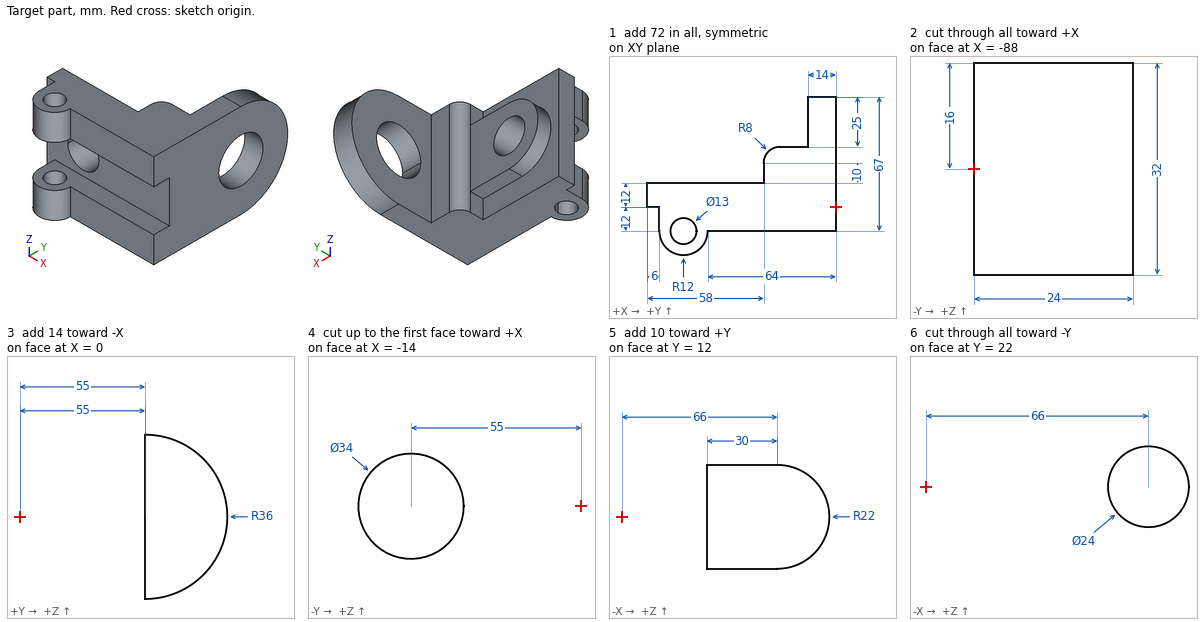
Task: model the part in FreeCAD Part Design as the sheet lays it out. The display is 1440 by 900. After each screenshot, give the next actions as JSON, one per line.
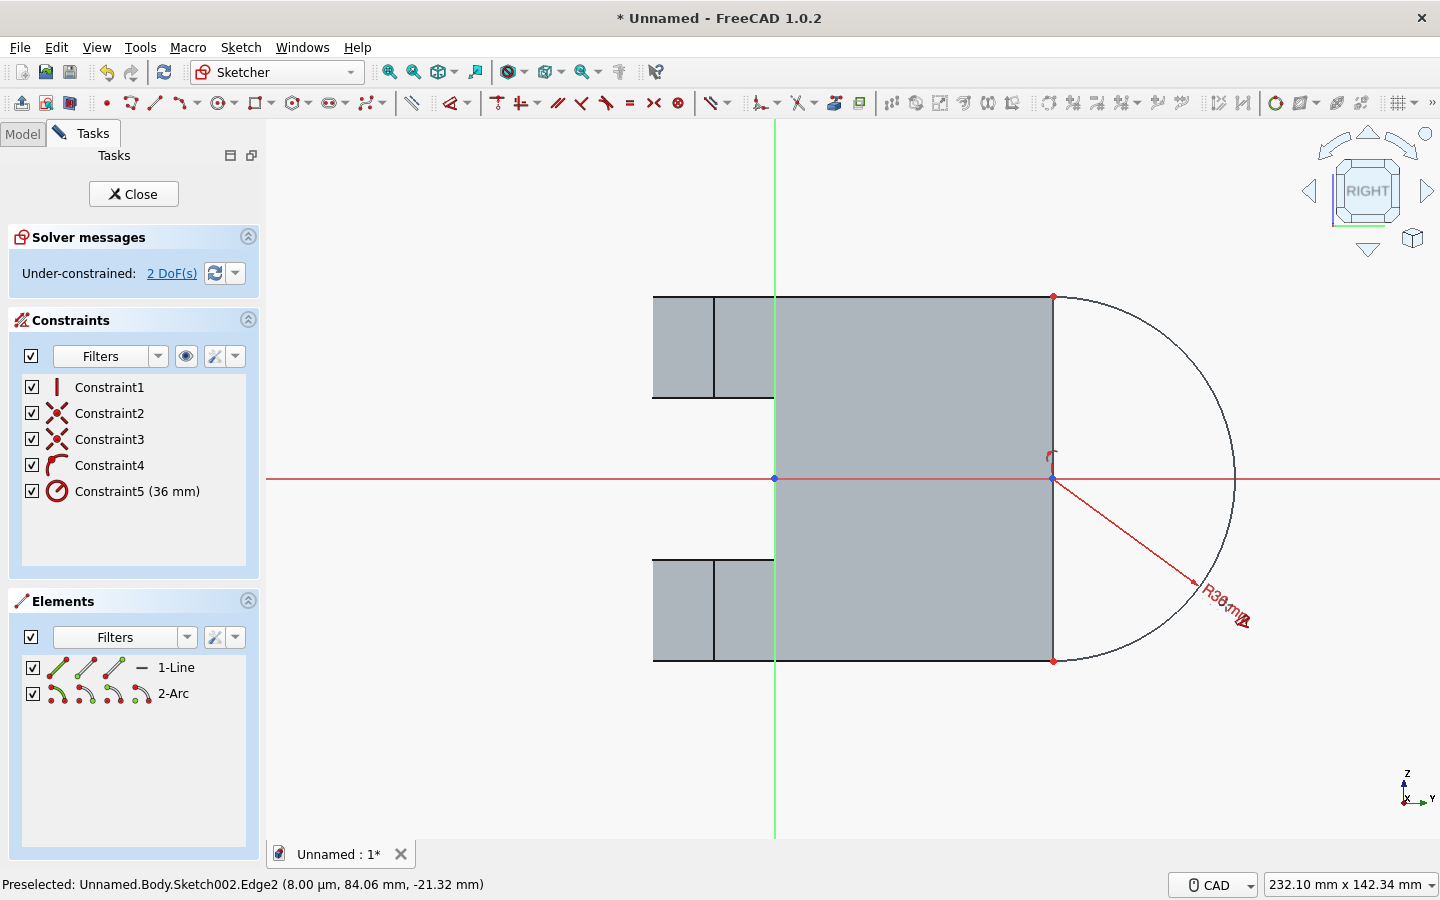
{"action": "left_click", "coordinate": [1053, 297]}
{"action": "left_click", "coordinate": [914, 263]}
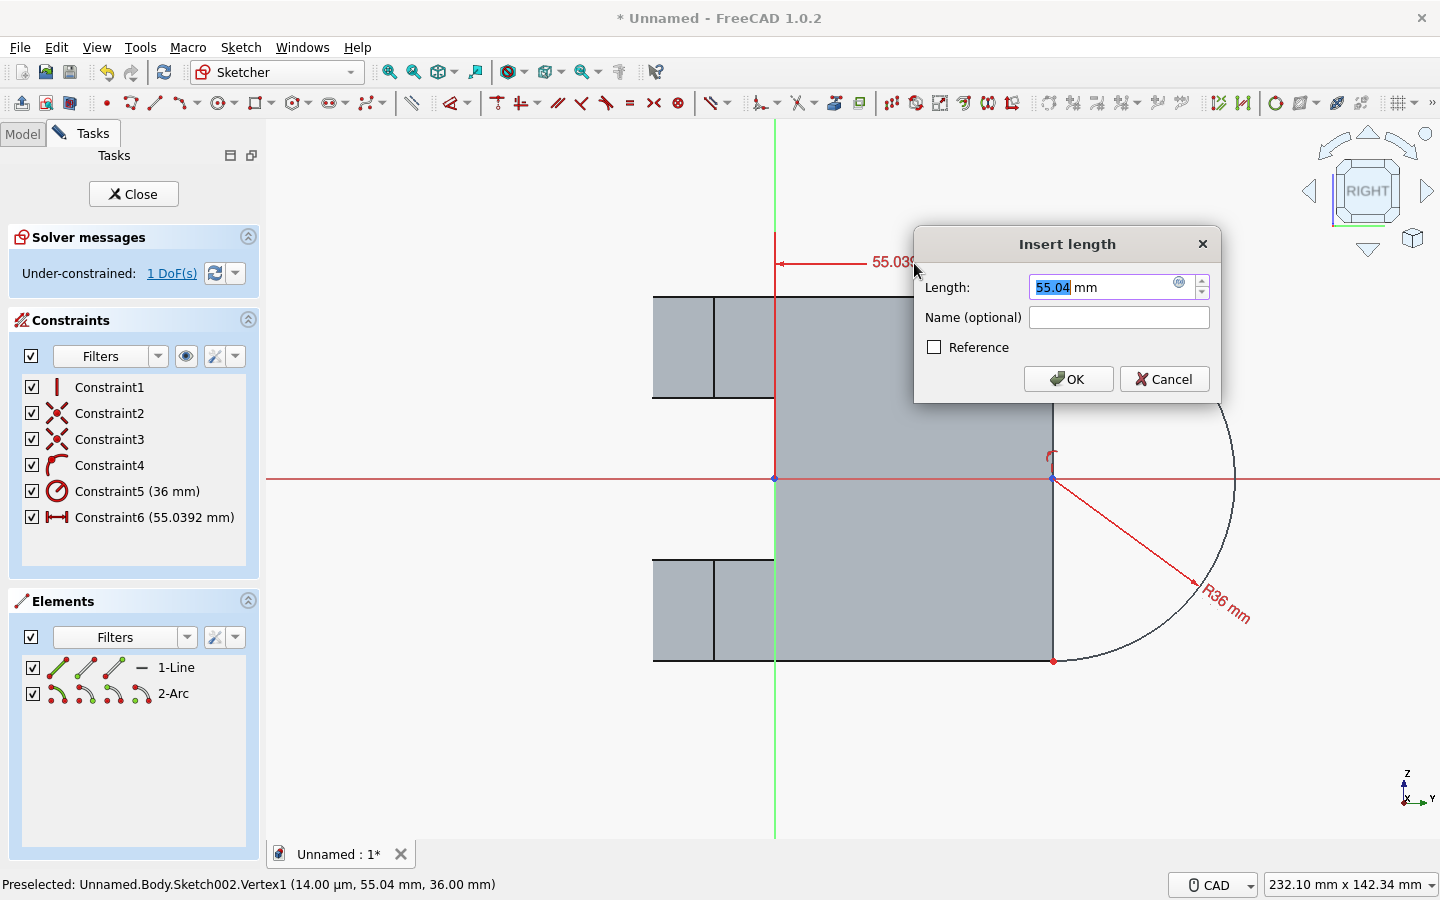
{"action": "type", "text": "55"}
{"action": "key", "text": "Return"}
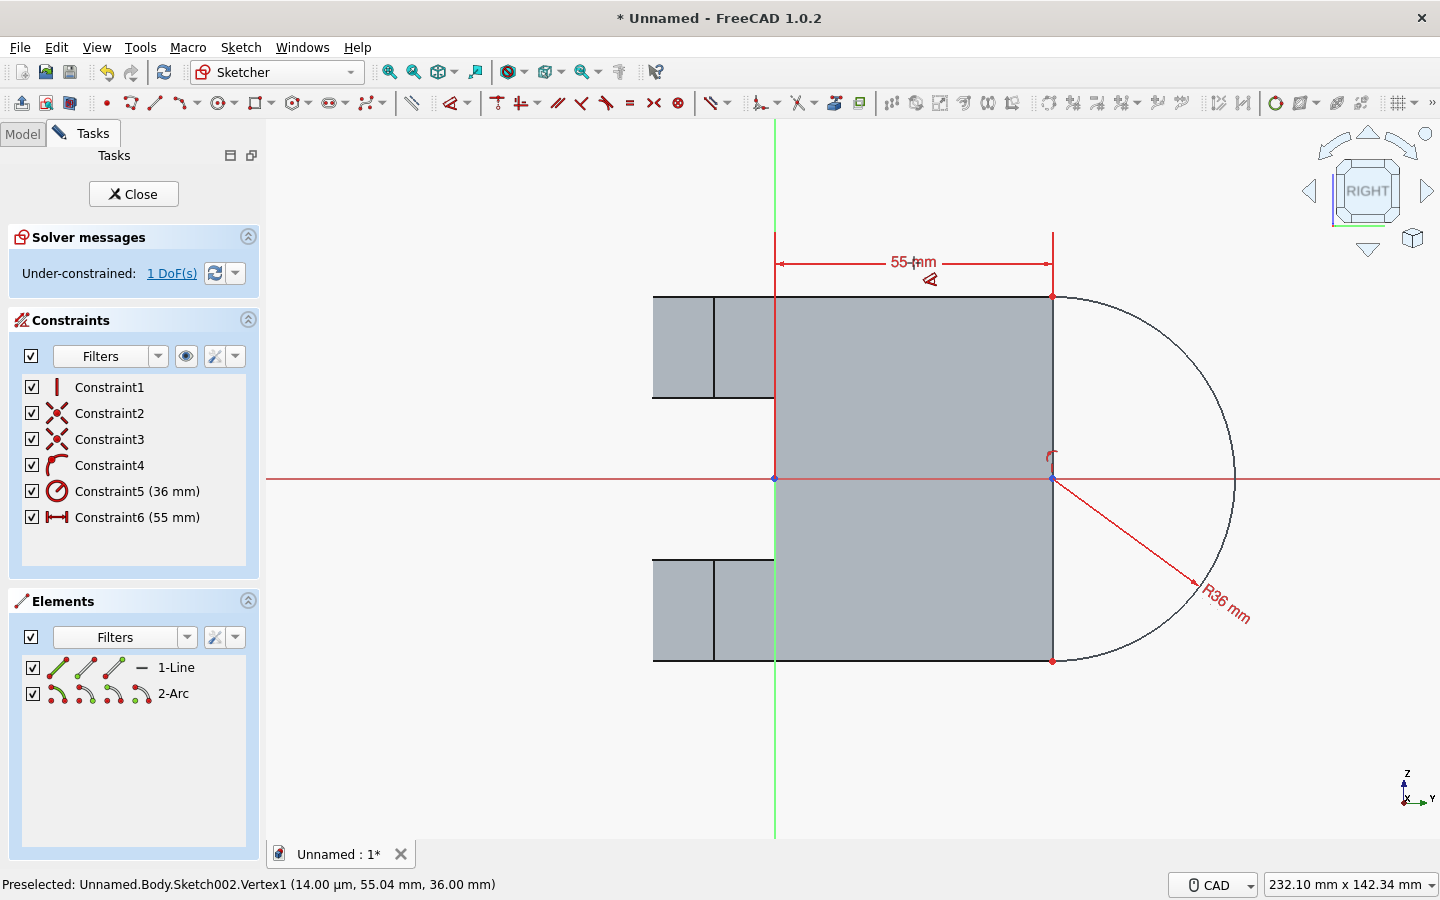
{"action": "left_click", "coordinate": [1053, 479]}
{"action": "left_click", "coordinate": [914, 513]}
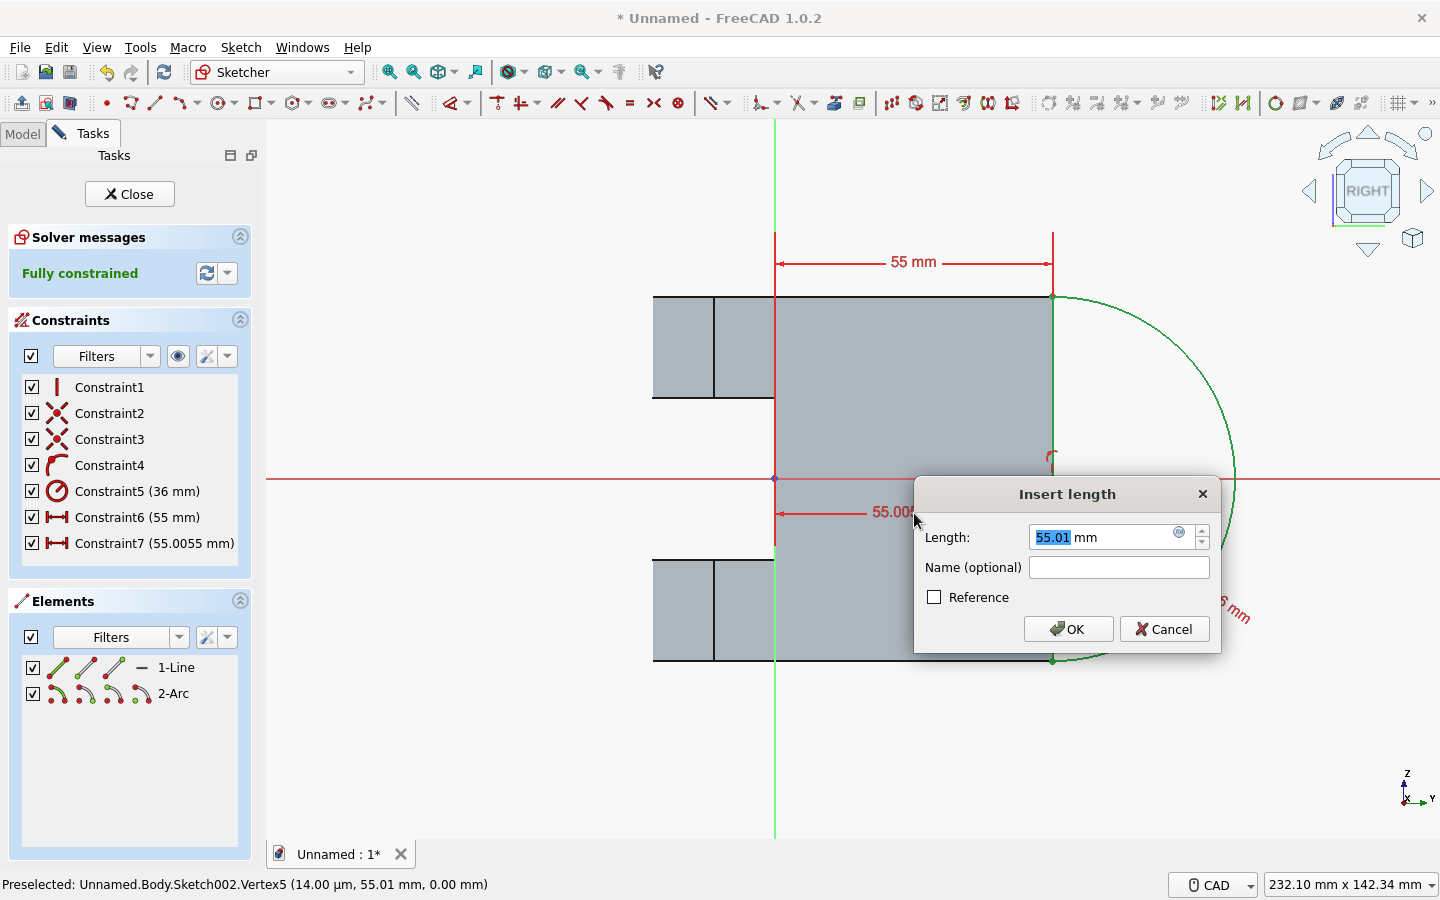
{"action": "type", "text": "55"}
{"action": "key", "text": "Return"}
{"action": "key", "text": "Escape"}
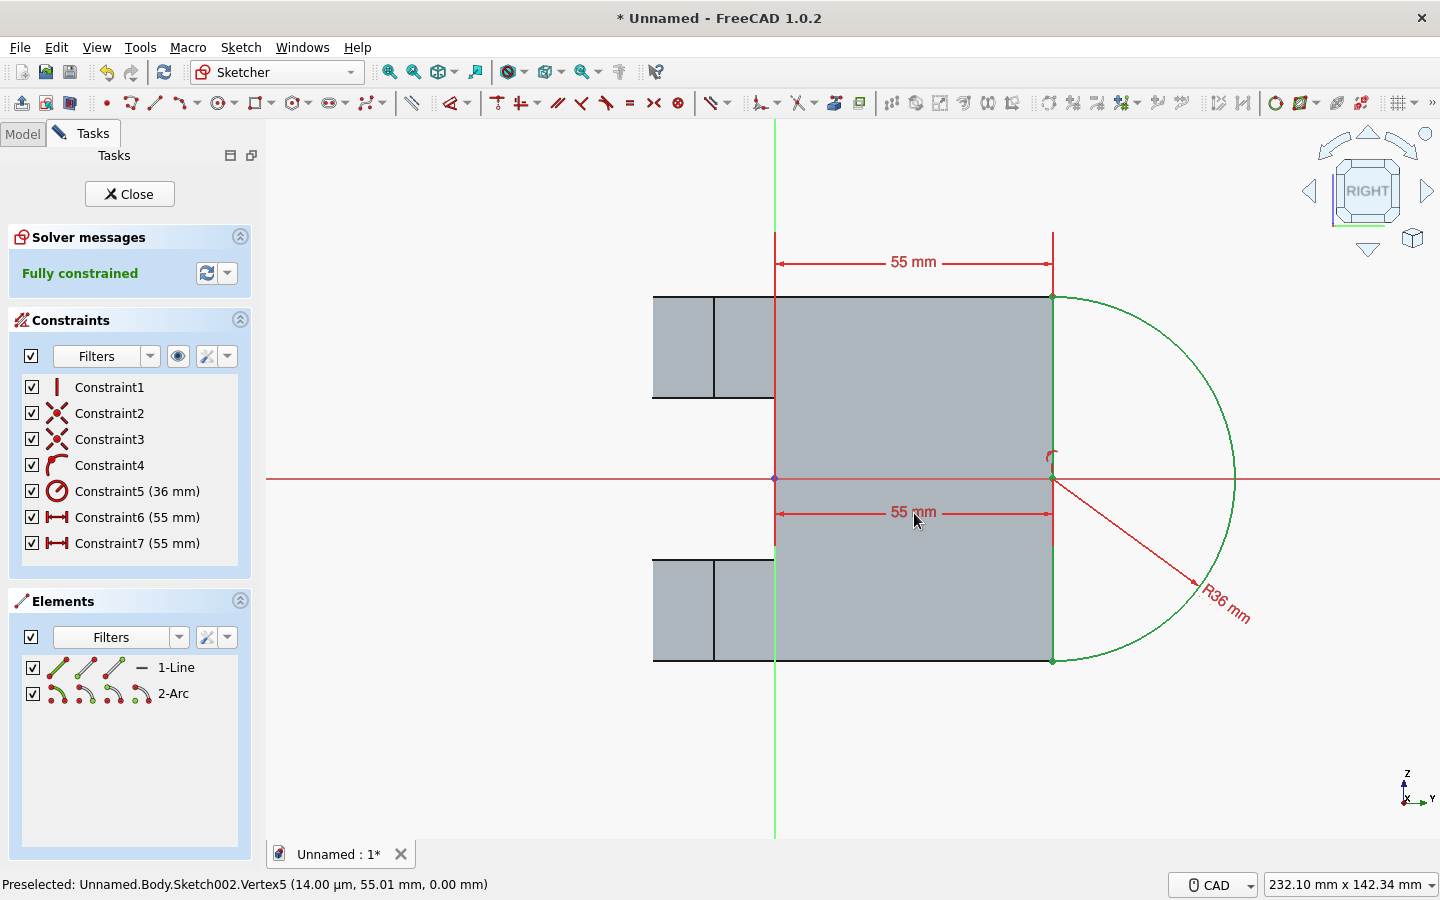
{"action": "left_click", "coordinate": [130, 194]}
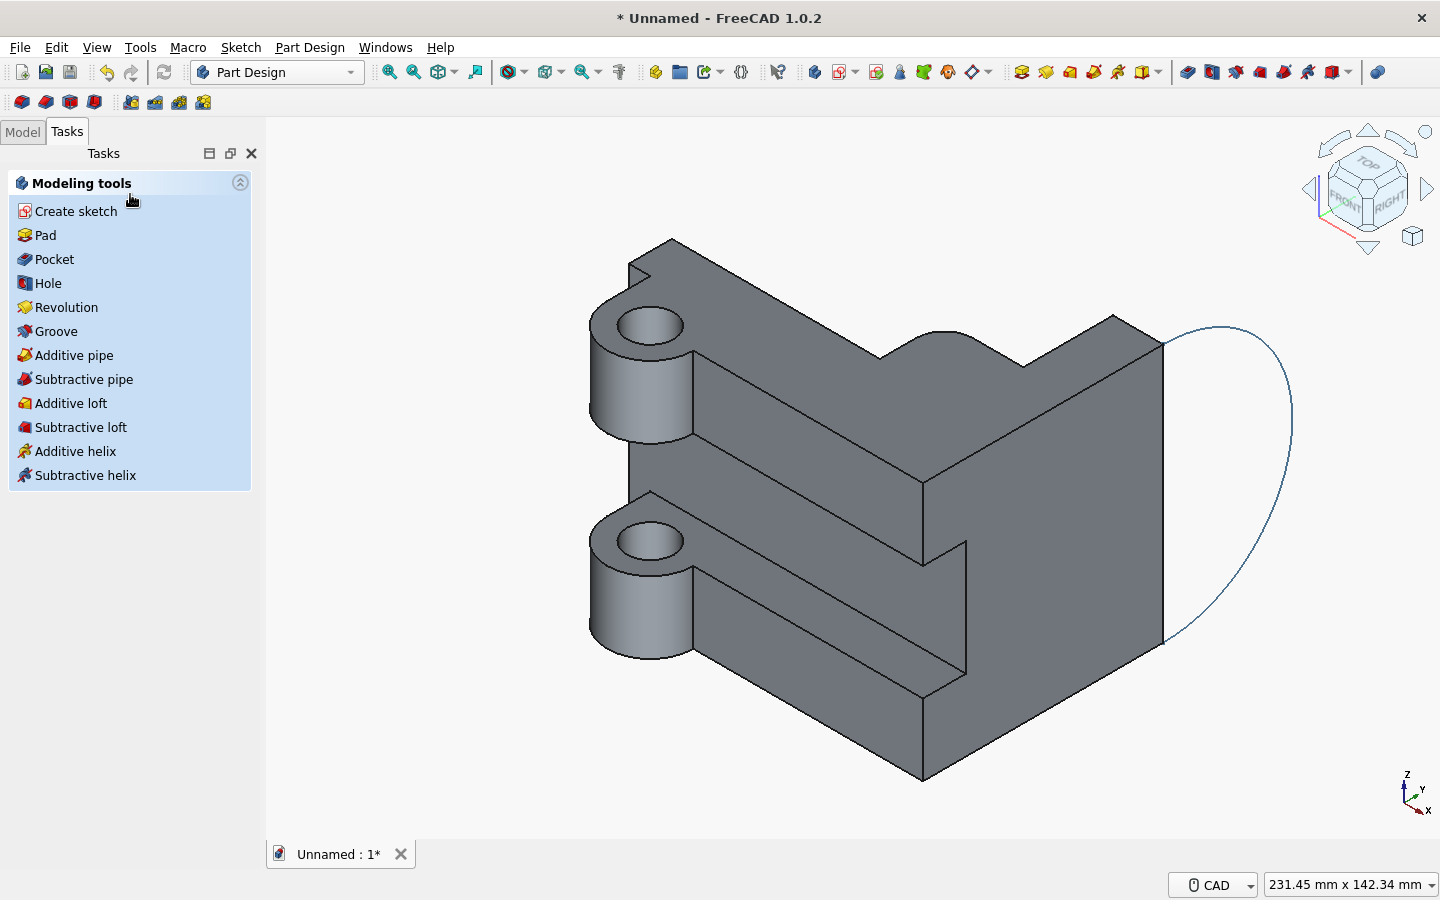
{"action": "left_click", "coordinate": [1022, 72]}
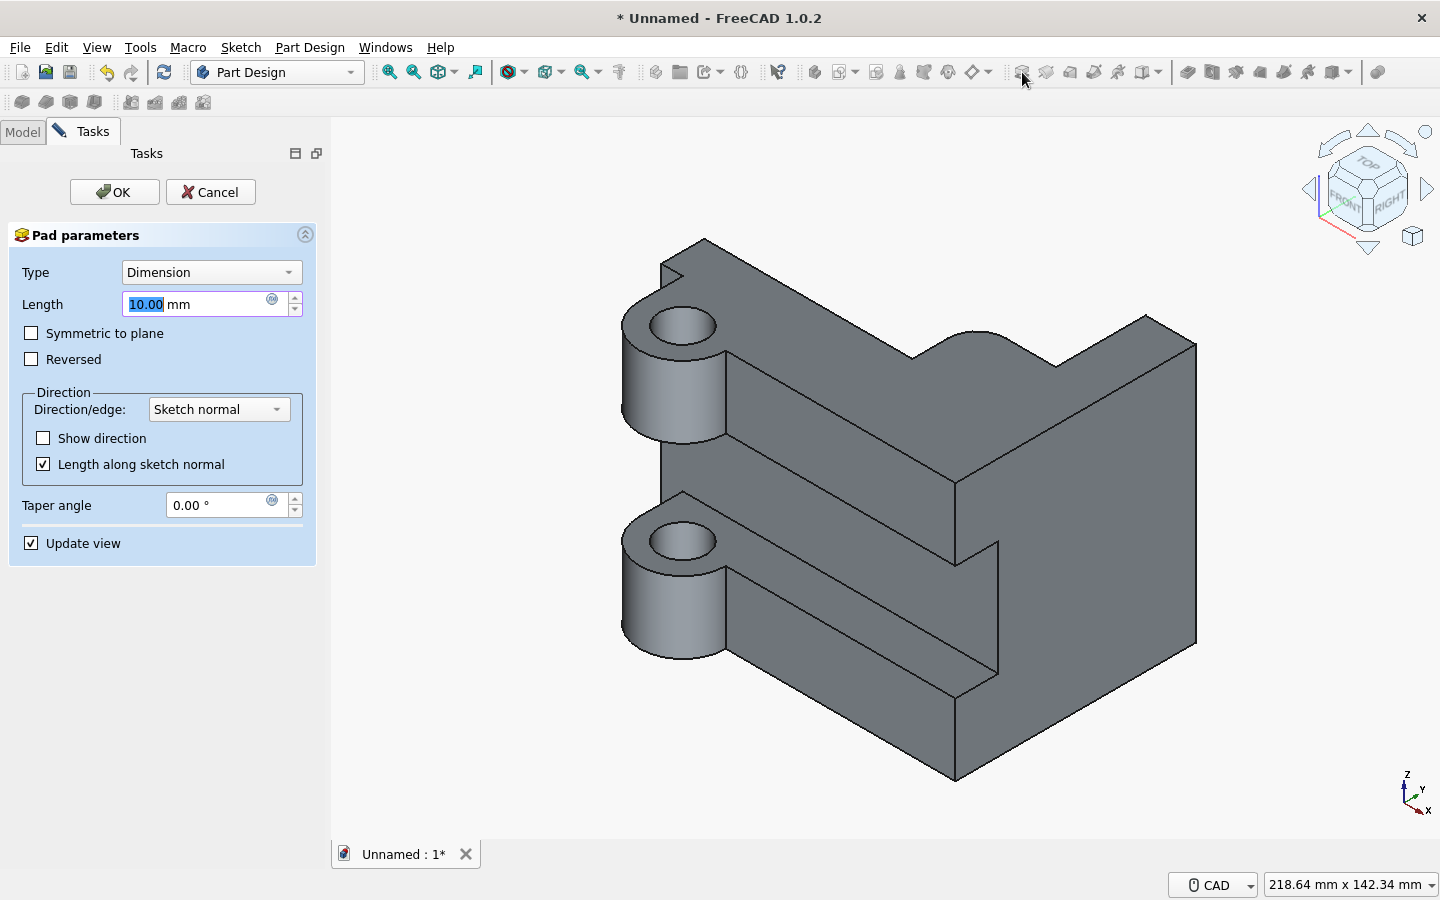
{"action": "type", "text": "14"}
{"action": "key", "text": "Tab"}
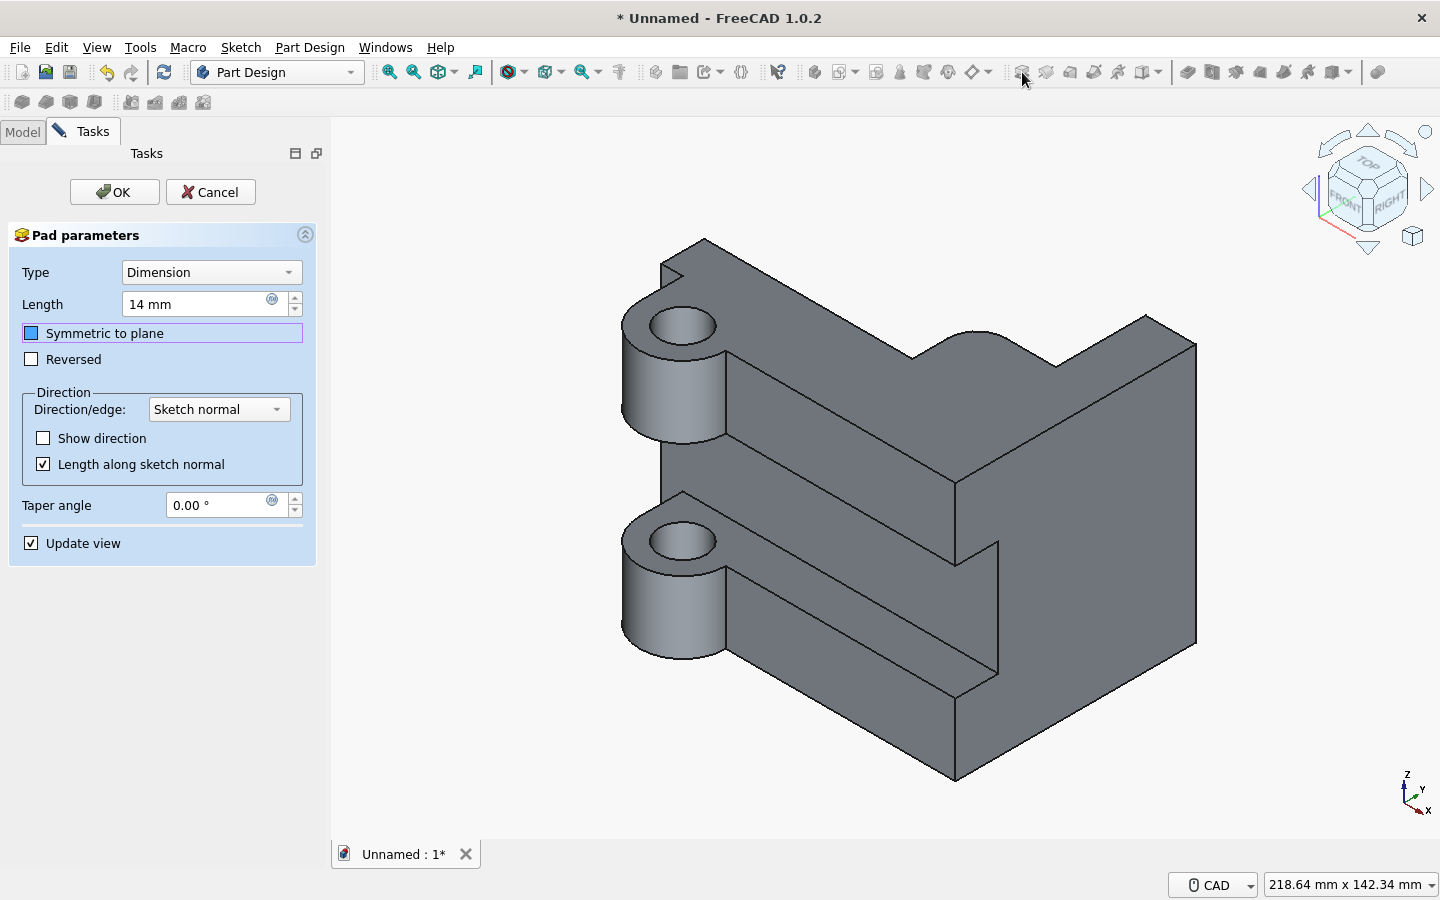
{"action": "left_click", "coordinate": [30, 359]}